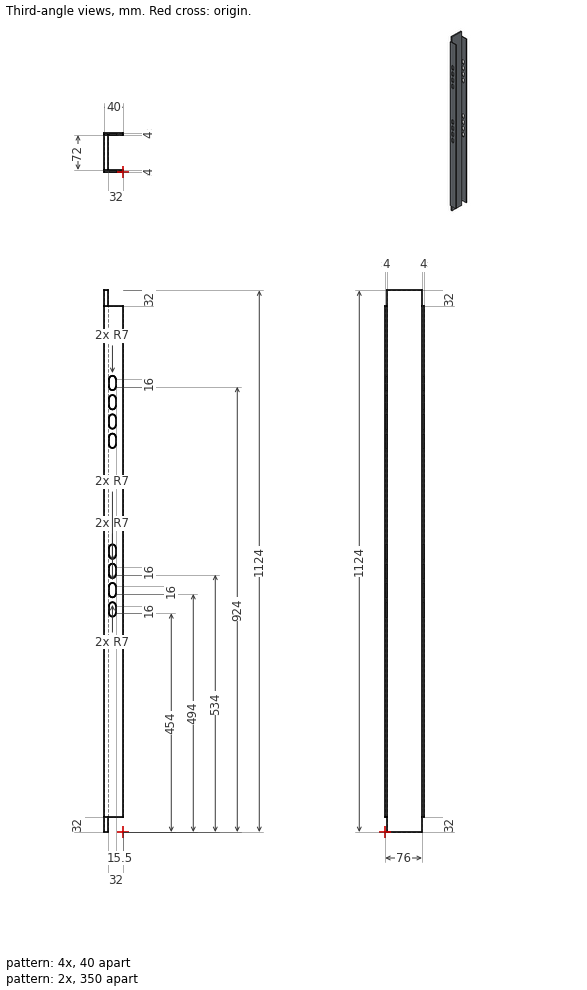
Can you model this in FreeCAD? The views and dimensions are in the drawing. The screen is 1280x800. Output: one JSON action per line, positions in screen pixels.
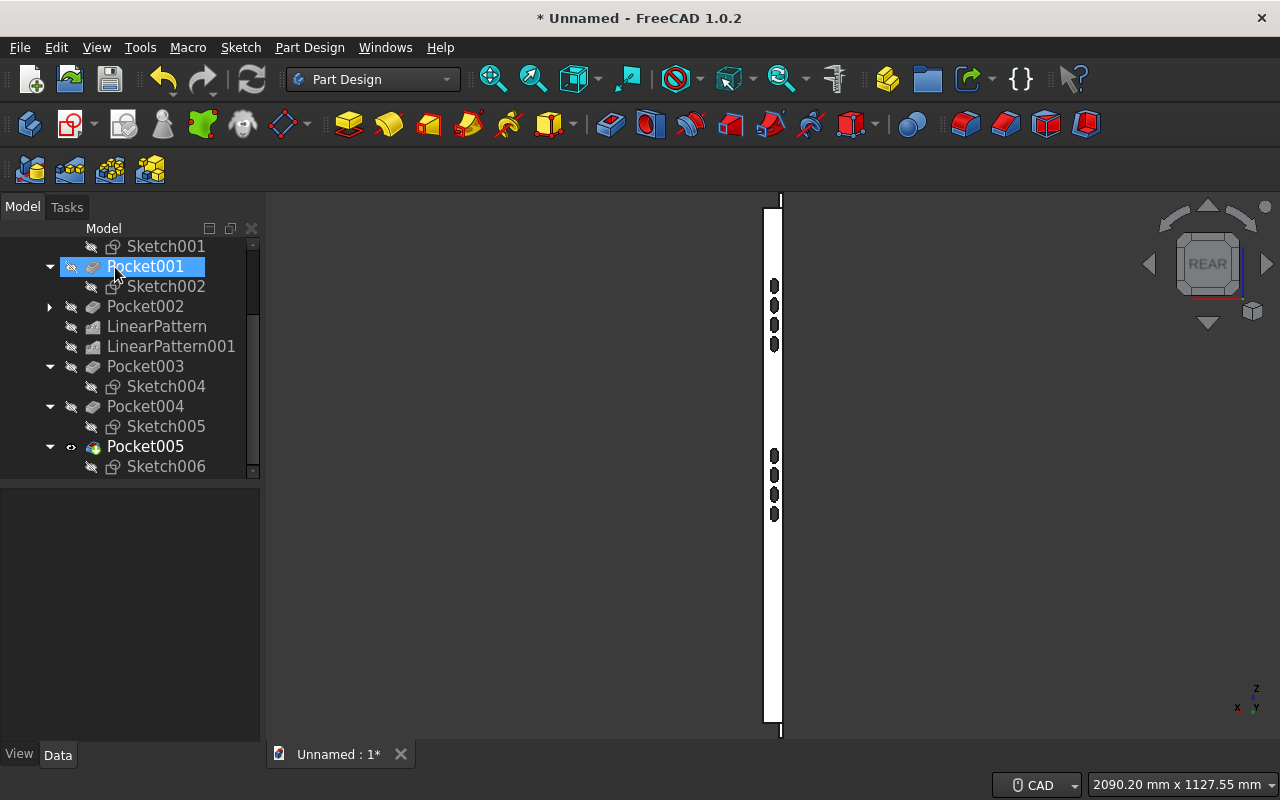
{"action": "key", "text": "0"}